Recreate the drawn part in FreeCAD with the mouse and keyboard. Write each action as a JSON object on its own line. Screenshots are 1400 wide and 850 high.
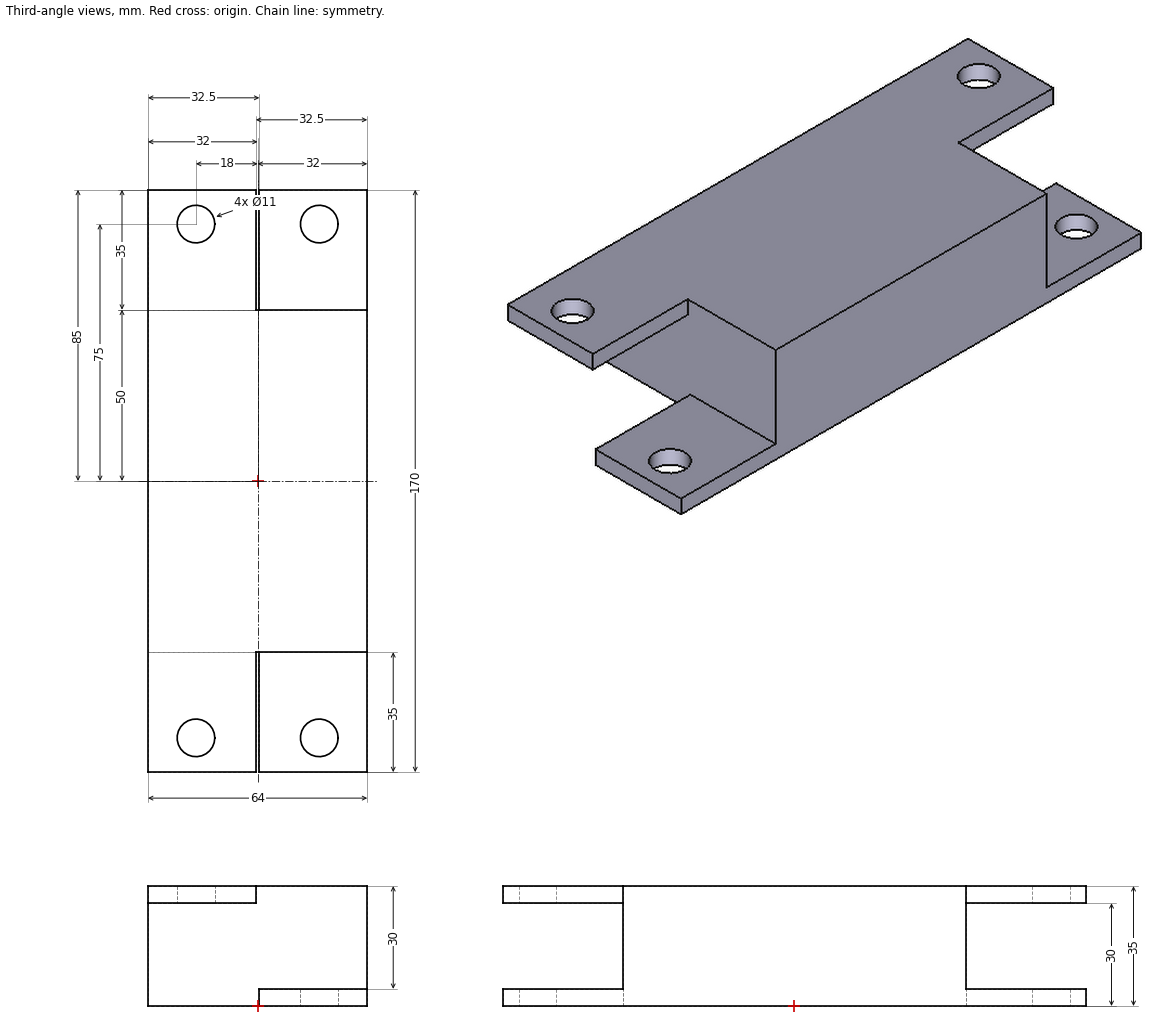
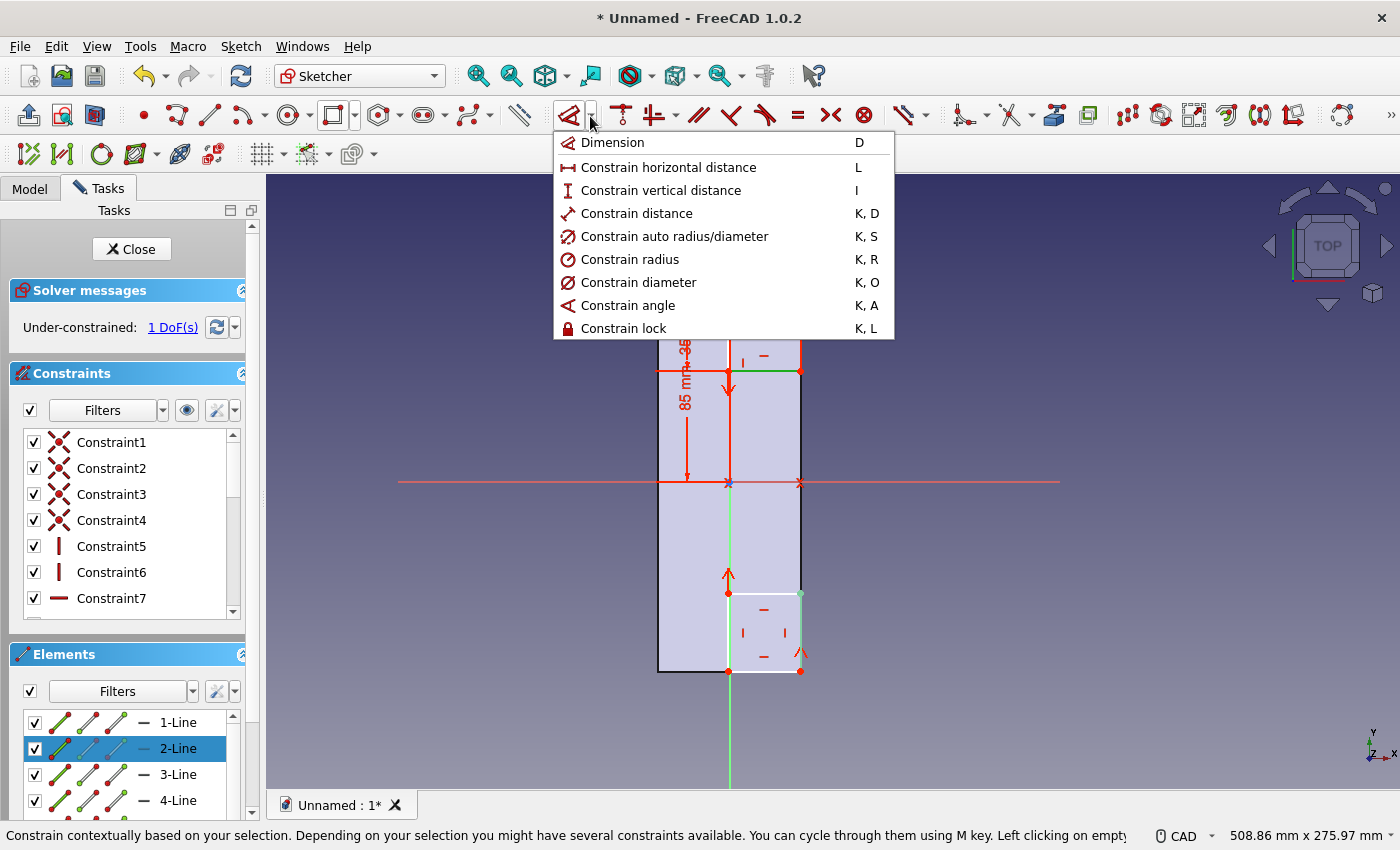
{"action": "left_click", "coordinate": [724, 168]}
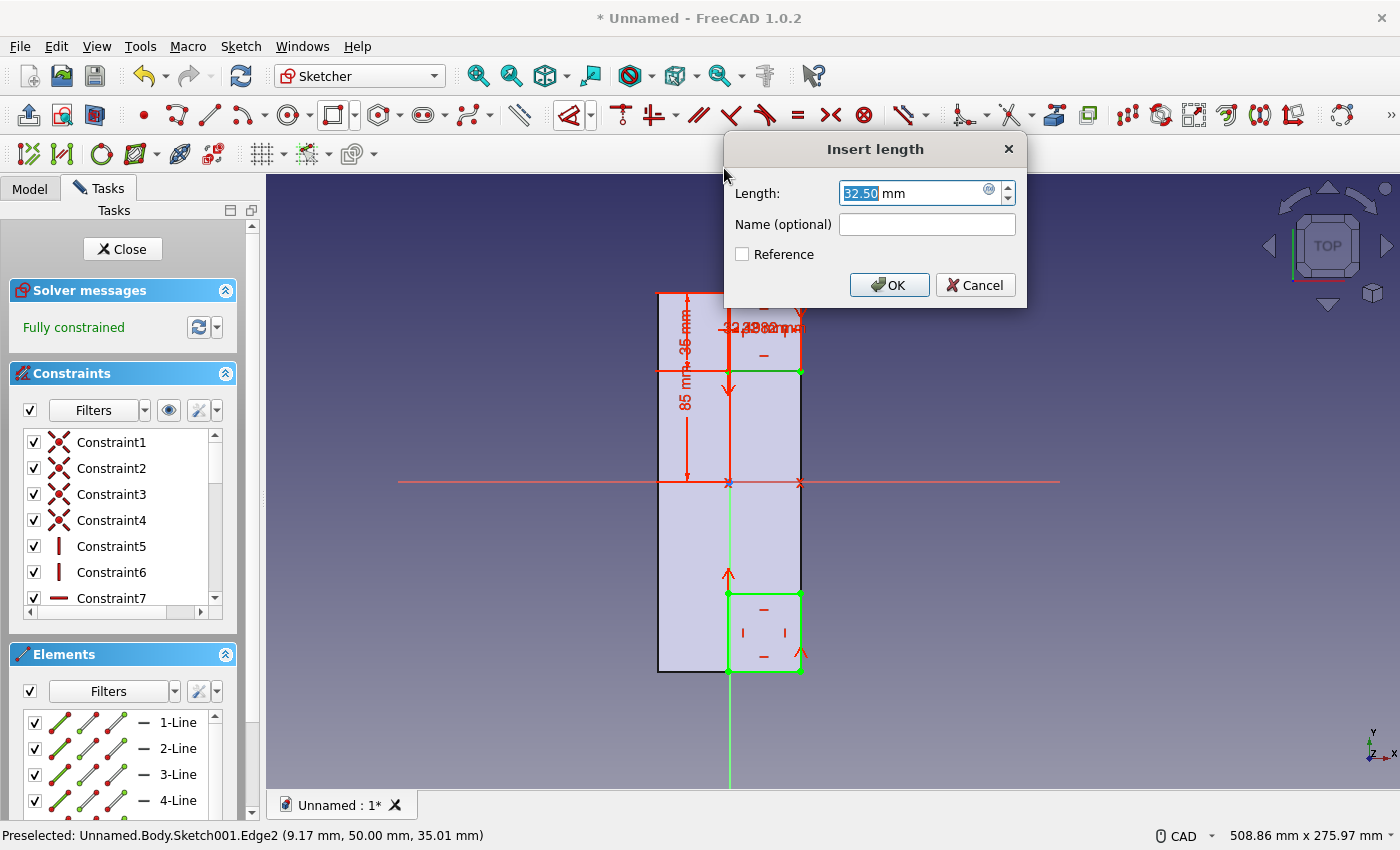
{"action": "type", "text": "32.5"}
{"action": "key", "text": "Return"}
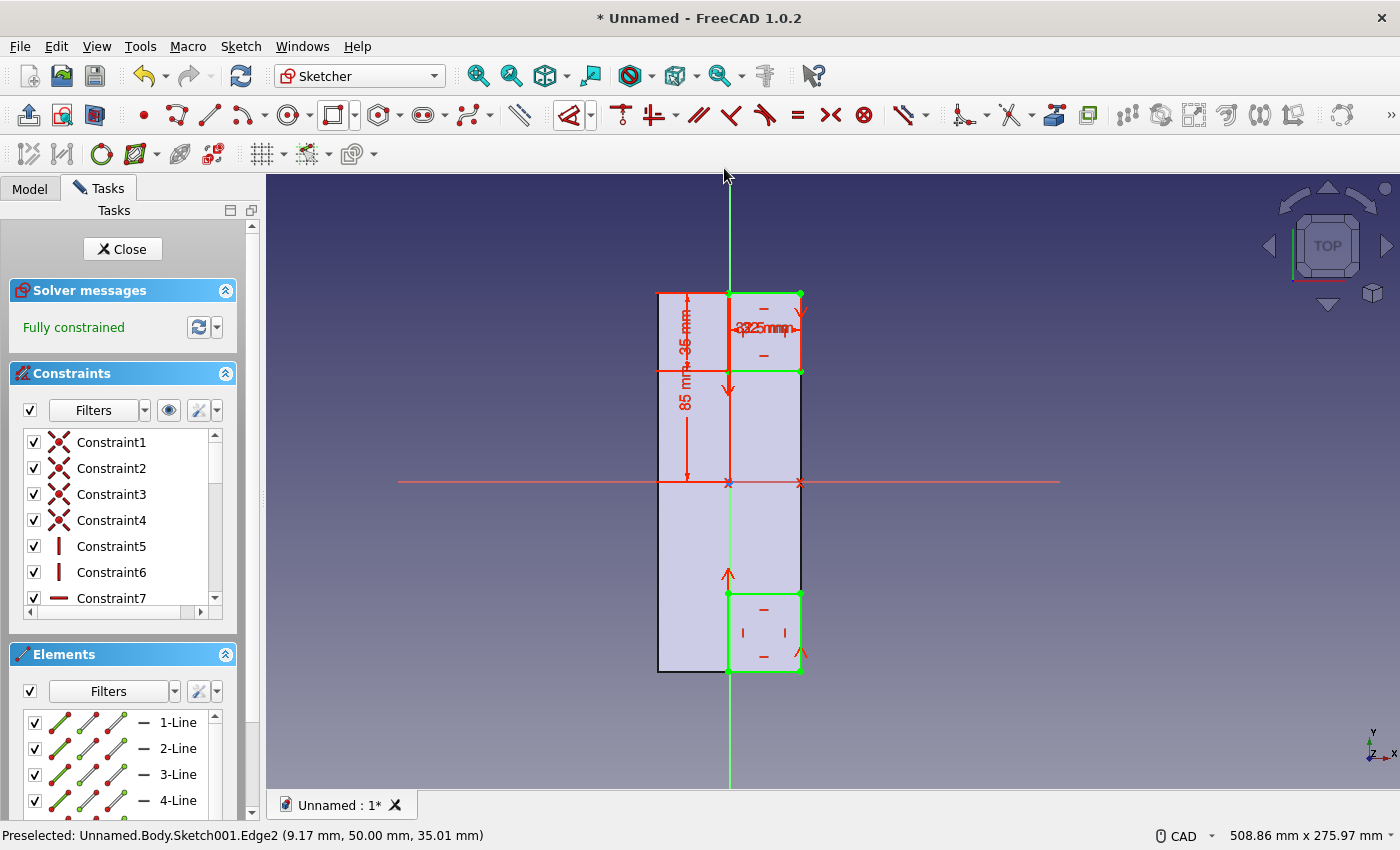
{"action": "left_click", "coordinate": [123, 249]}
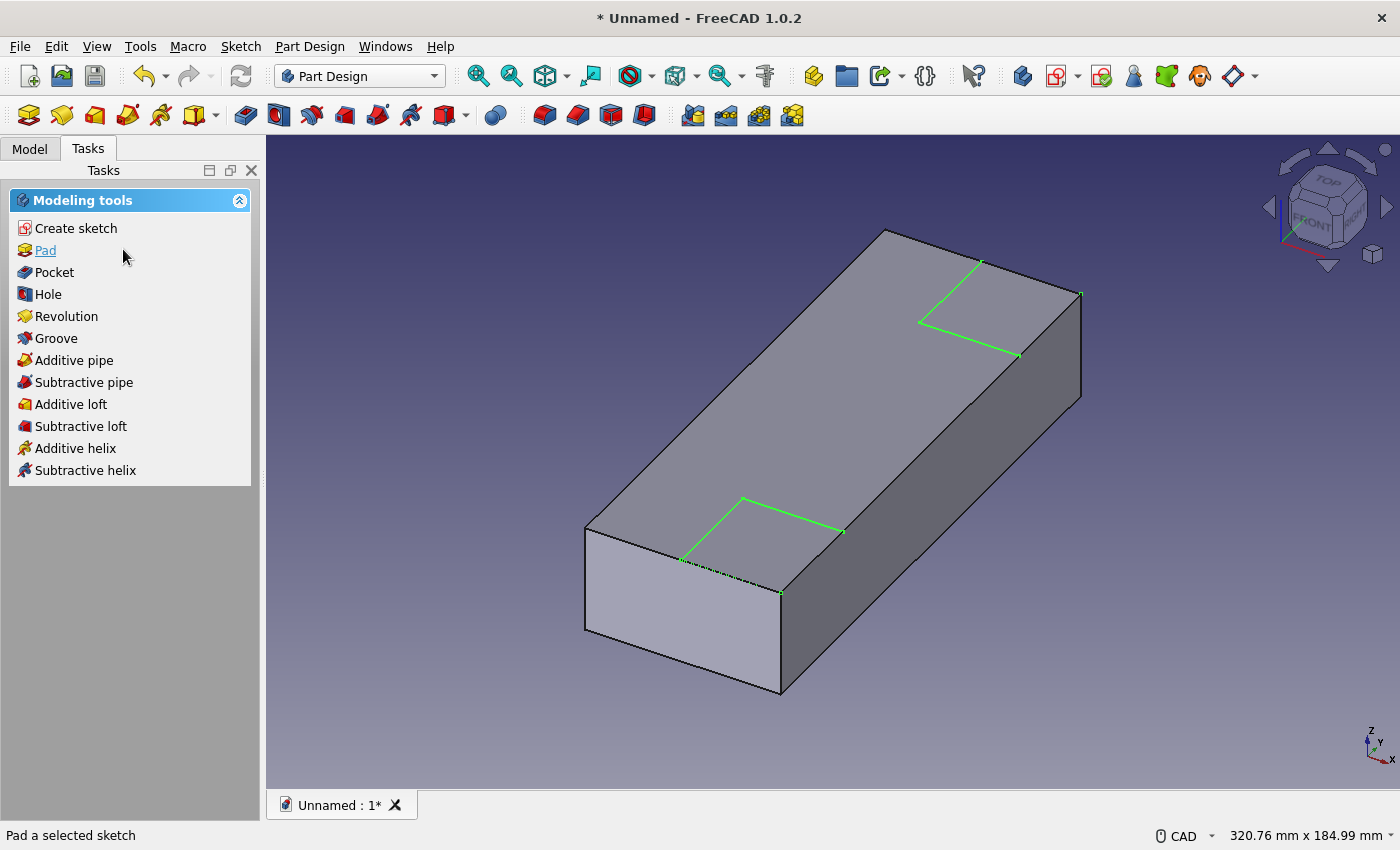
{"action": "left_click", "coordinate": [246, 116]}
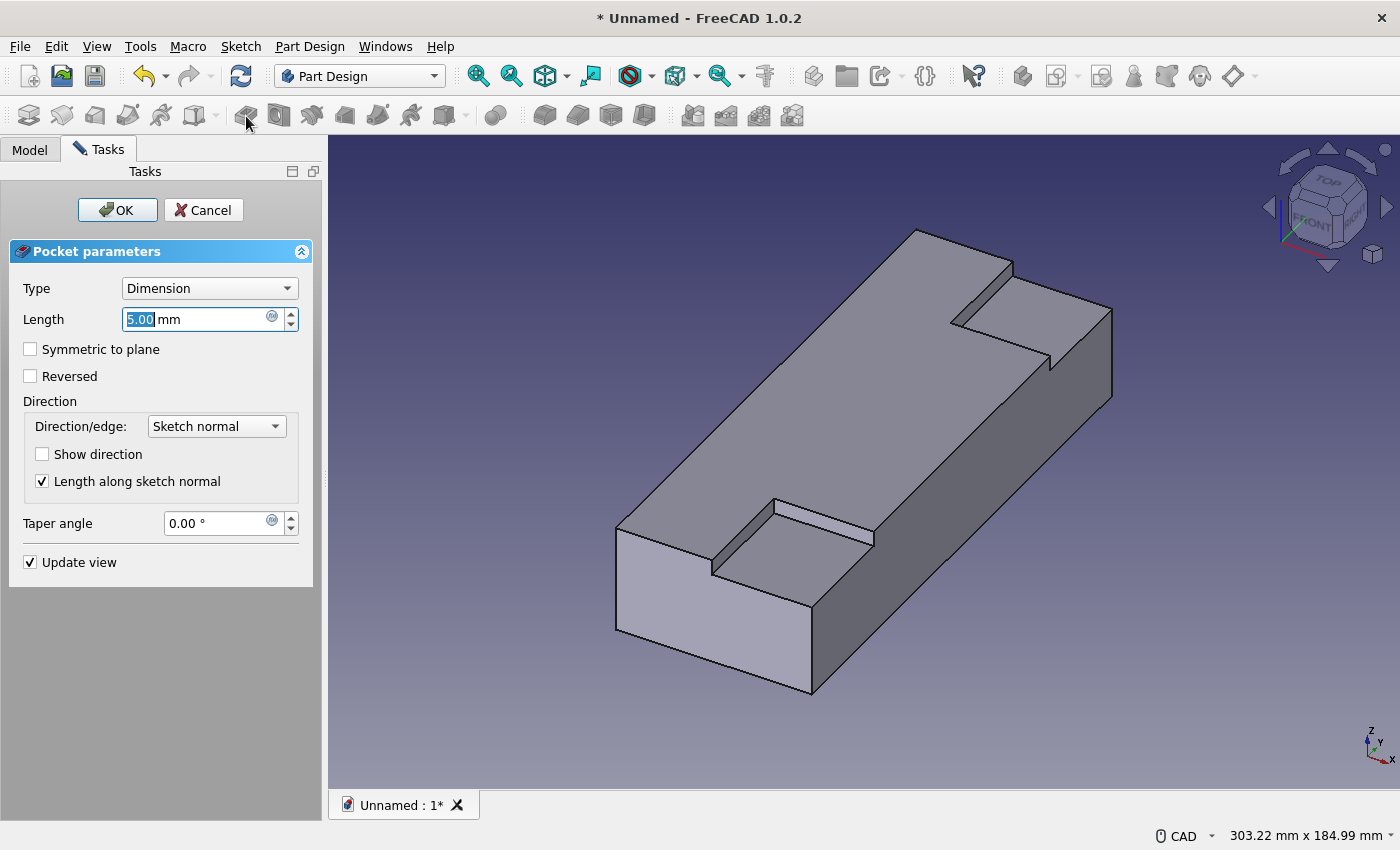
{"action": "type", "text": "30"}
{"action": "key", "text": "Tab"}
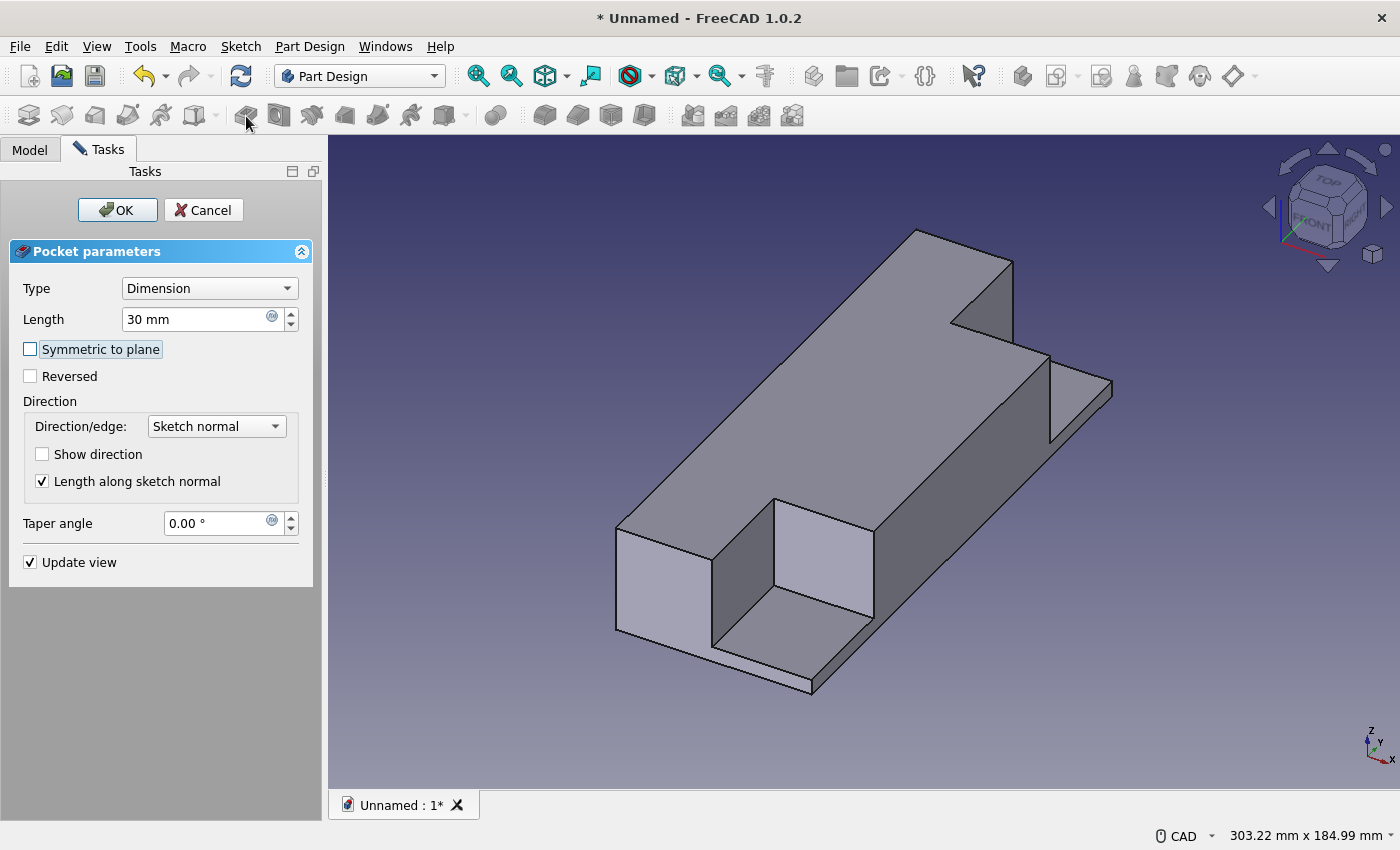
{"action": "left_click", "coordinate": [118, 210]}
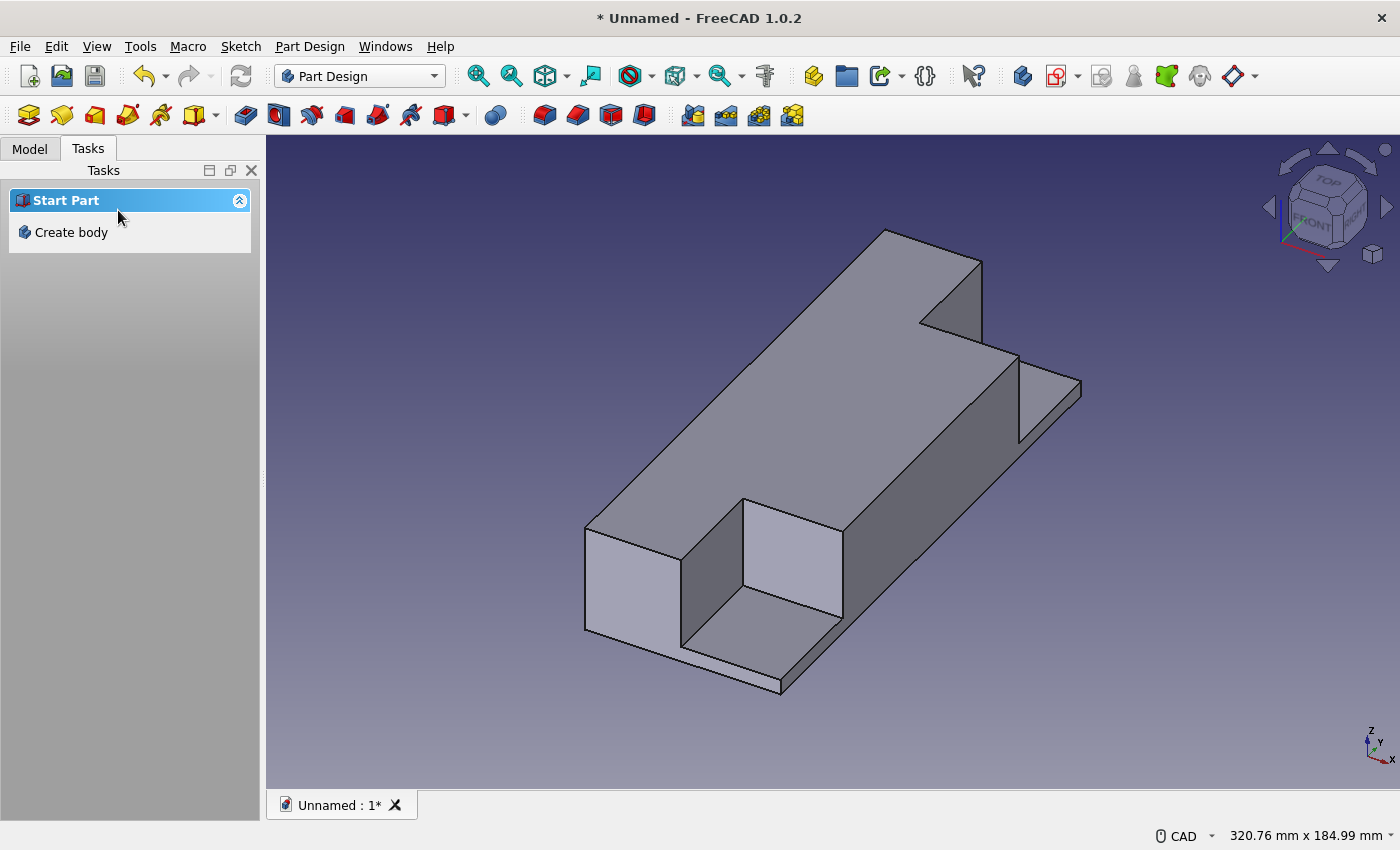
{"action": "key", "text": "5"}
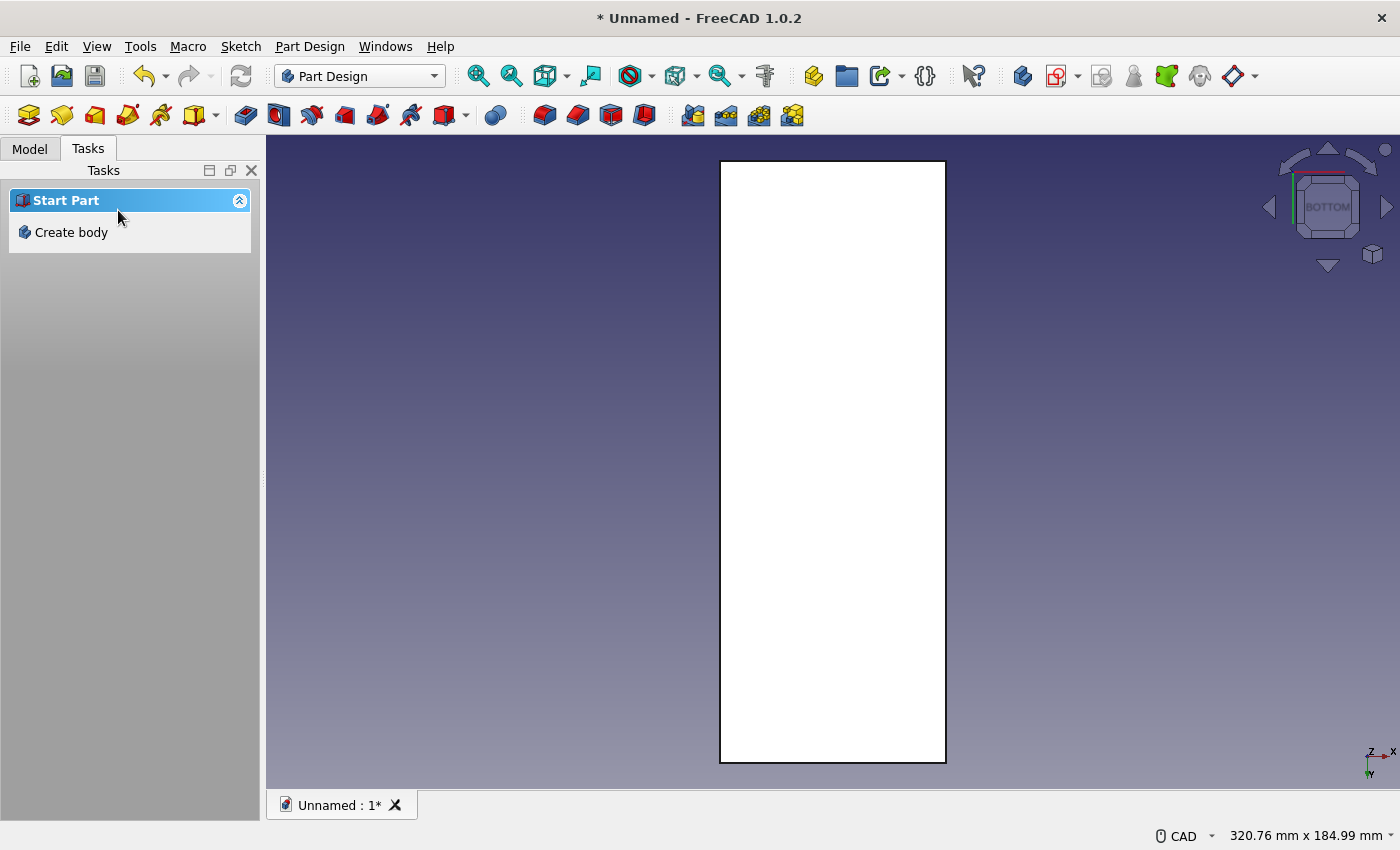
{"action": "left_click", "coordinate": [833, 633]}